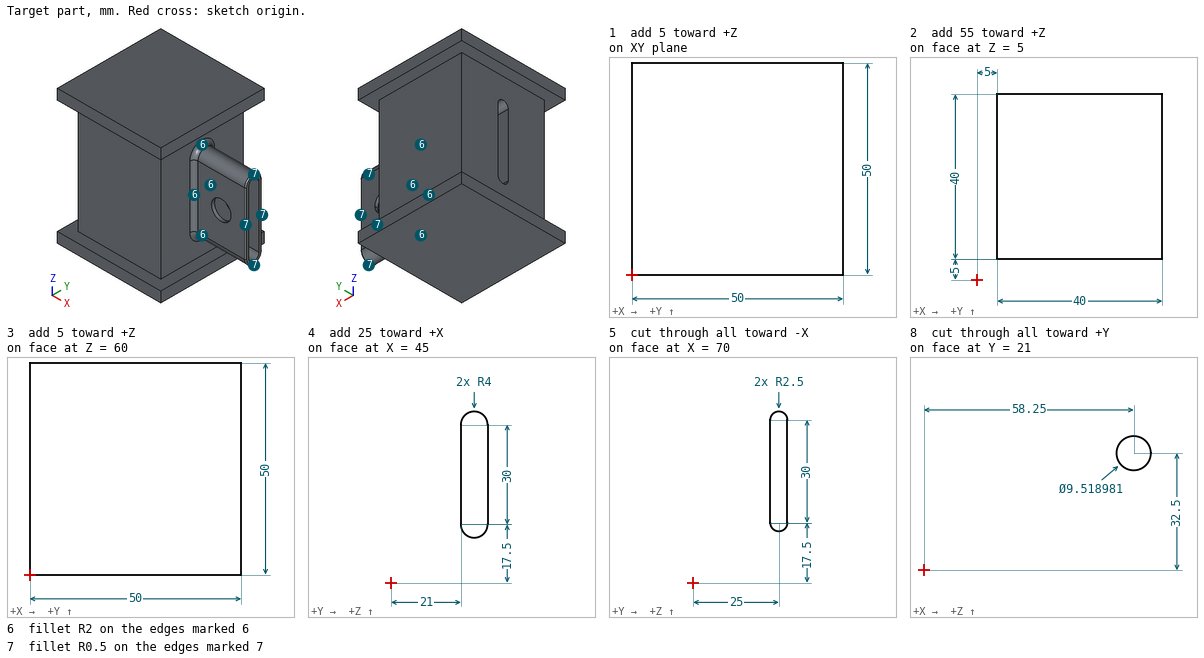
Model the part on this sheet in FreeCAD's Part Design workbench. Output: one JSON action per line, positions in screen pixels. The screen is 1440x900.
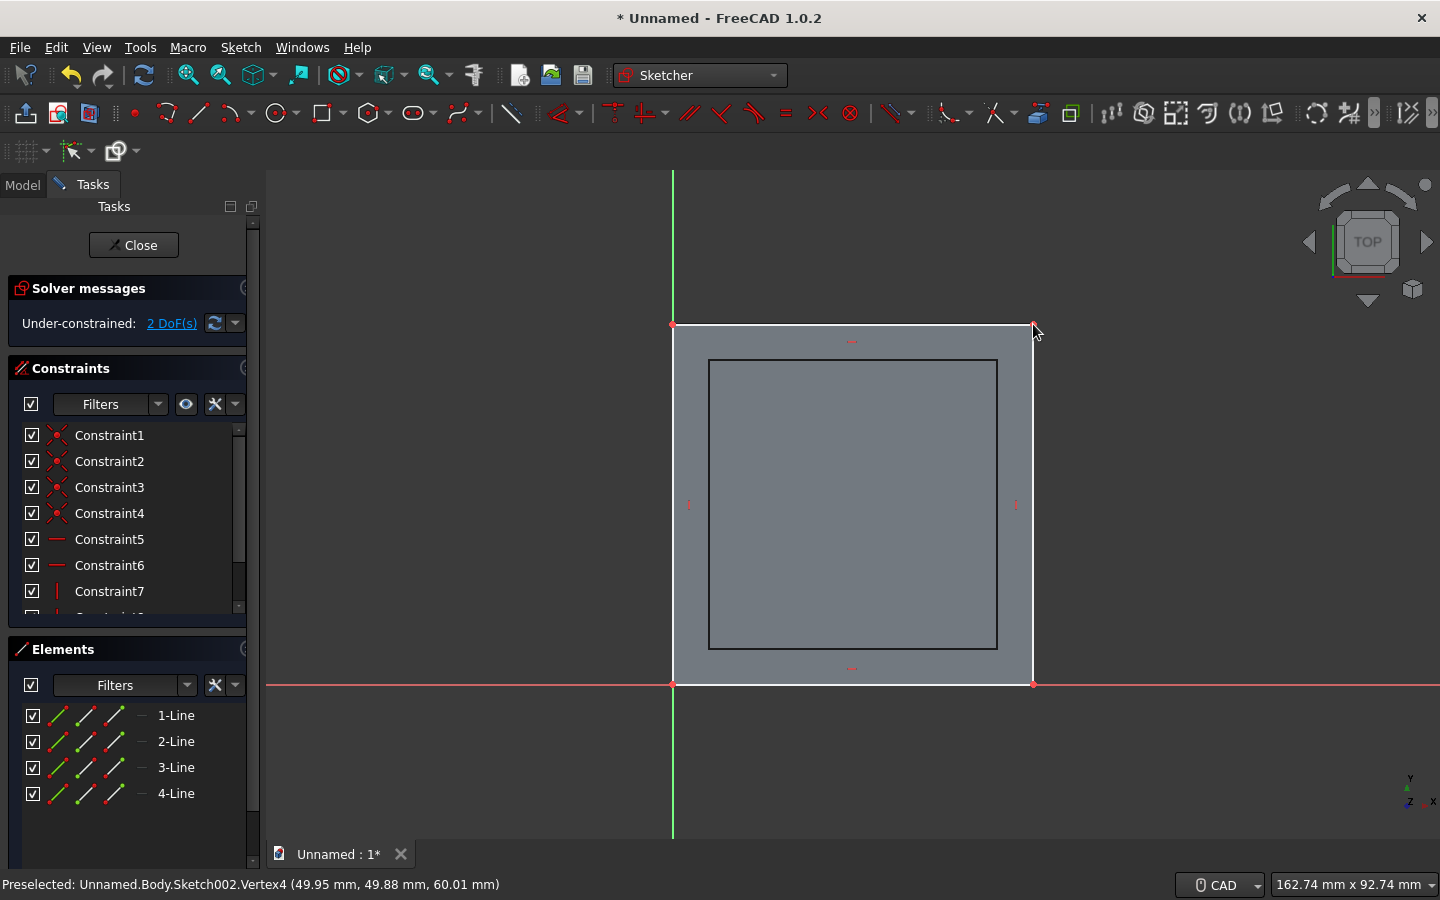
{"action": "left_click", "coordinate": [558, 114]}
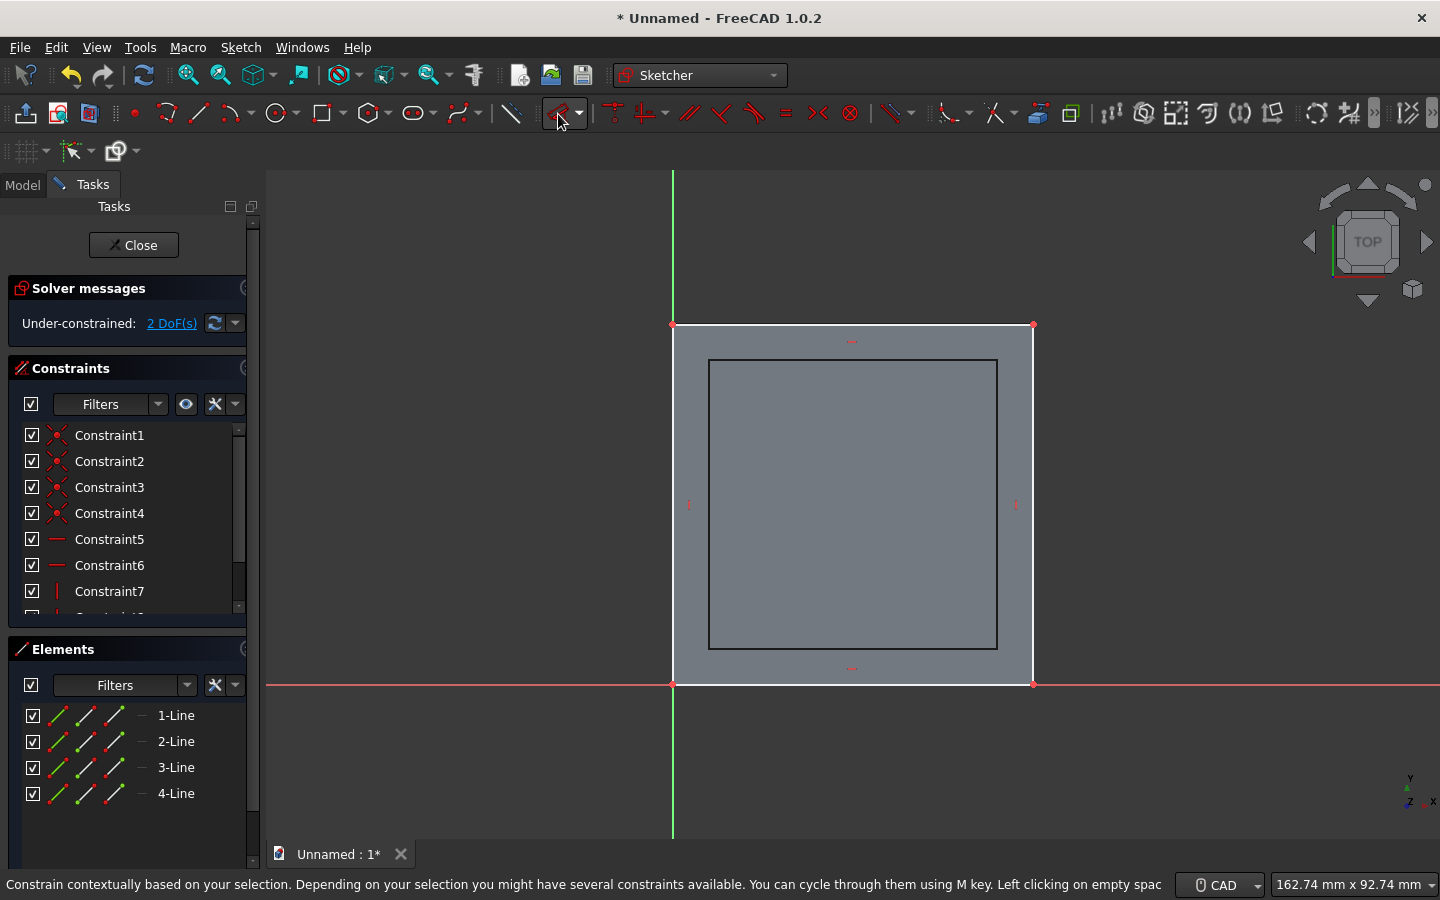
{"action": "left_click", "coordinate": [781, 685]}
{"action": "left_click", "coordinate": [853, 719]}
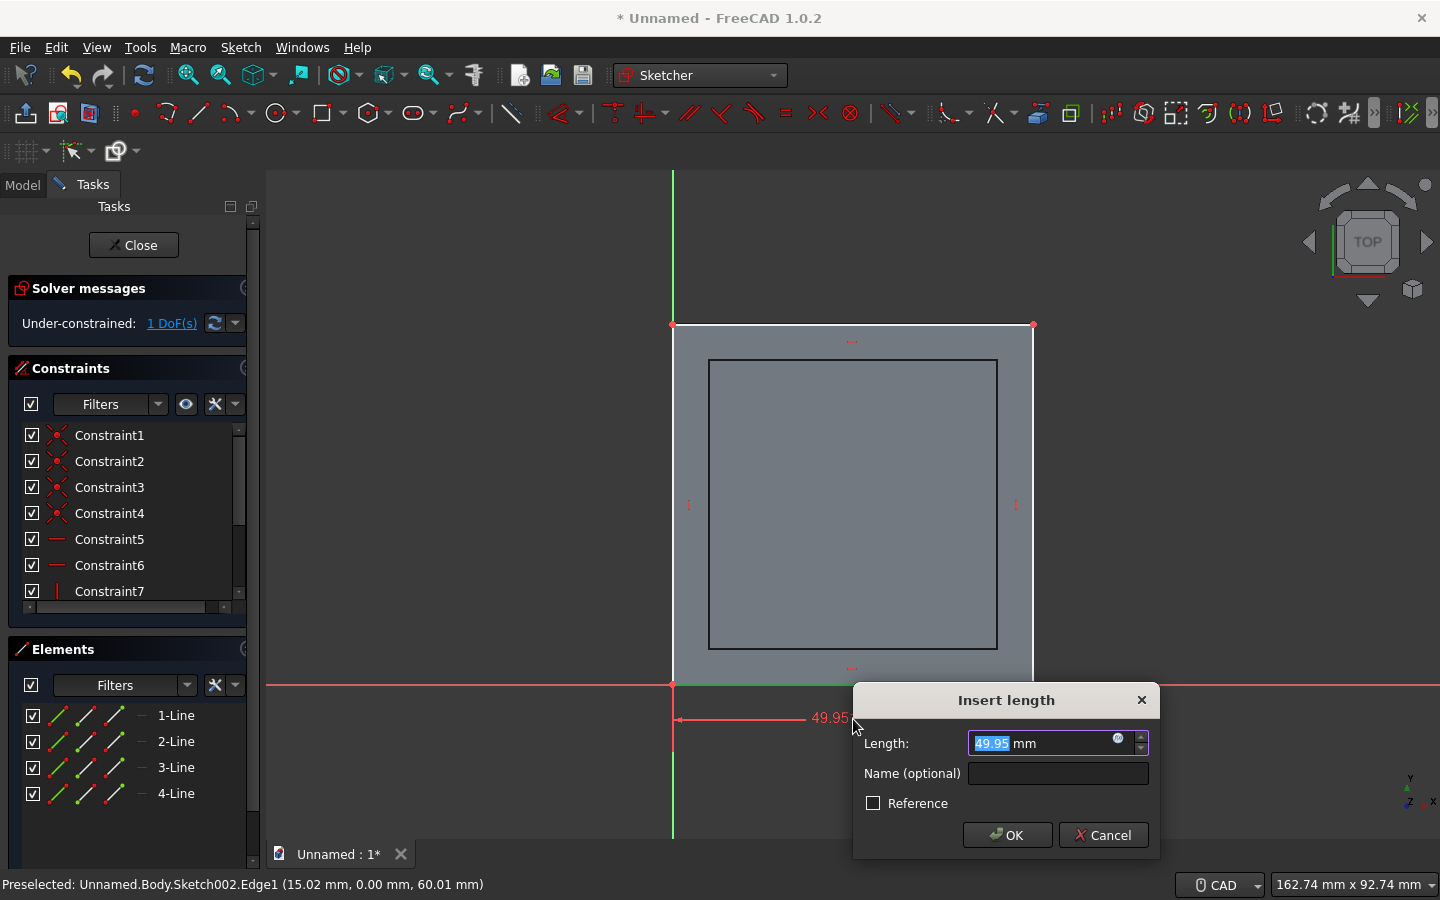
{"action": "type", "text": "50"}
{"action": "key", "text": "Return"}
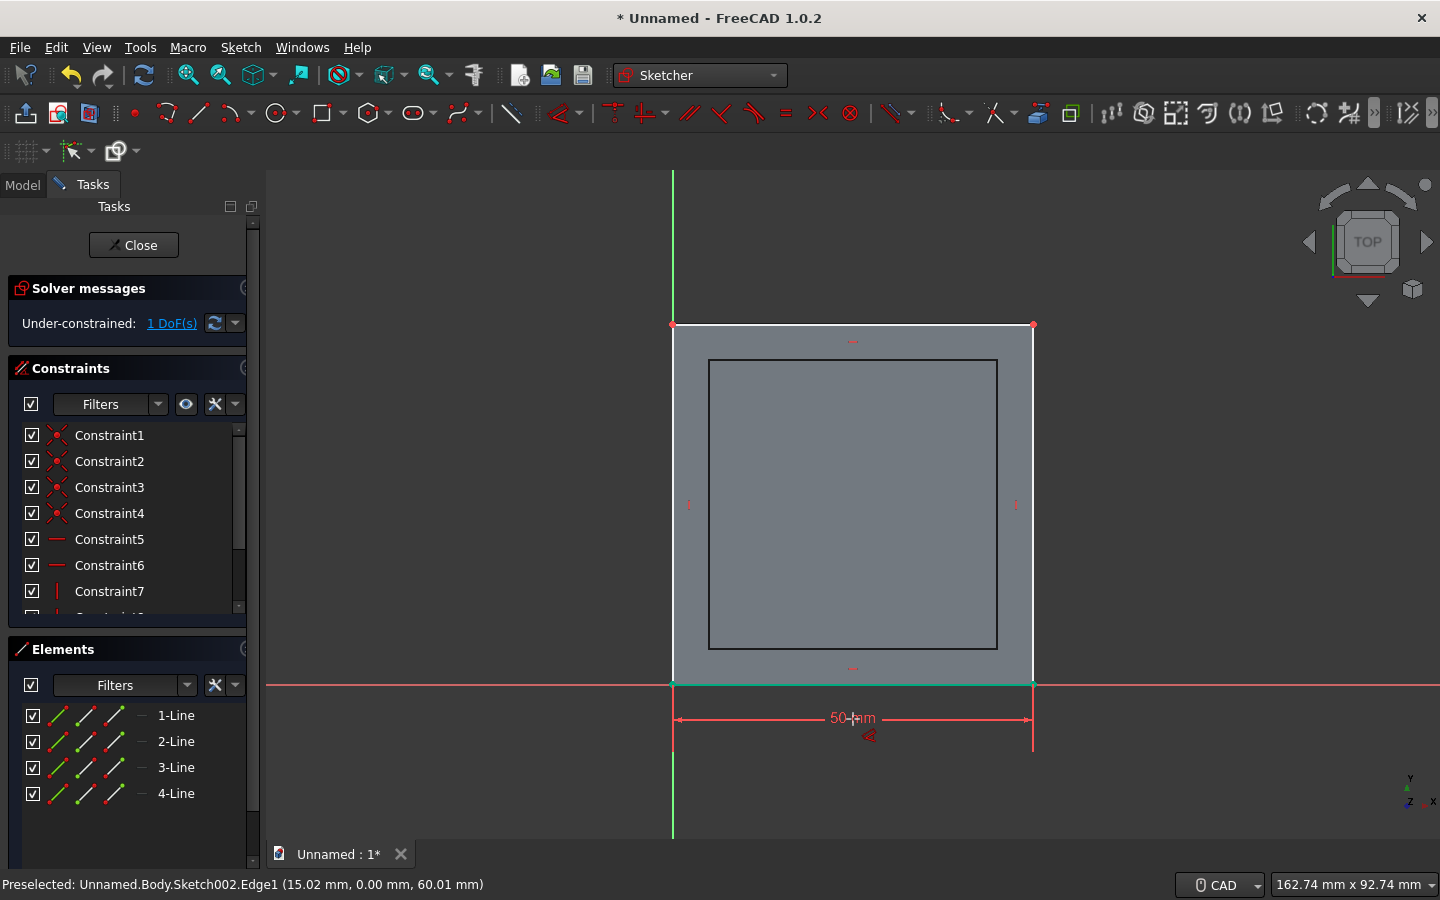
{"action": "left_click", "coordinate": [1033, 577]}
{"action": "left_click", "coordinate": [1067, 505]}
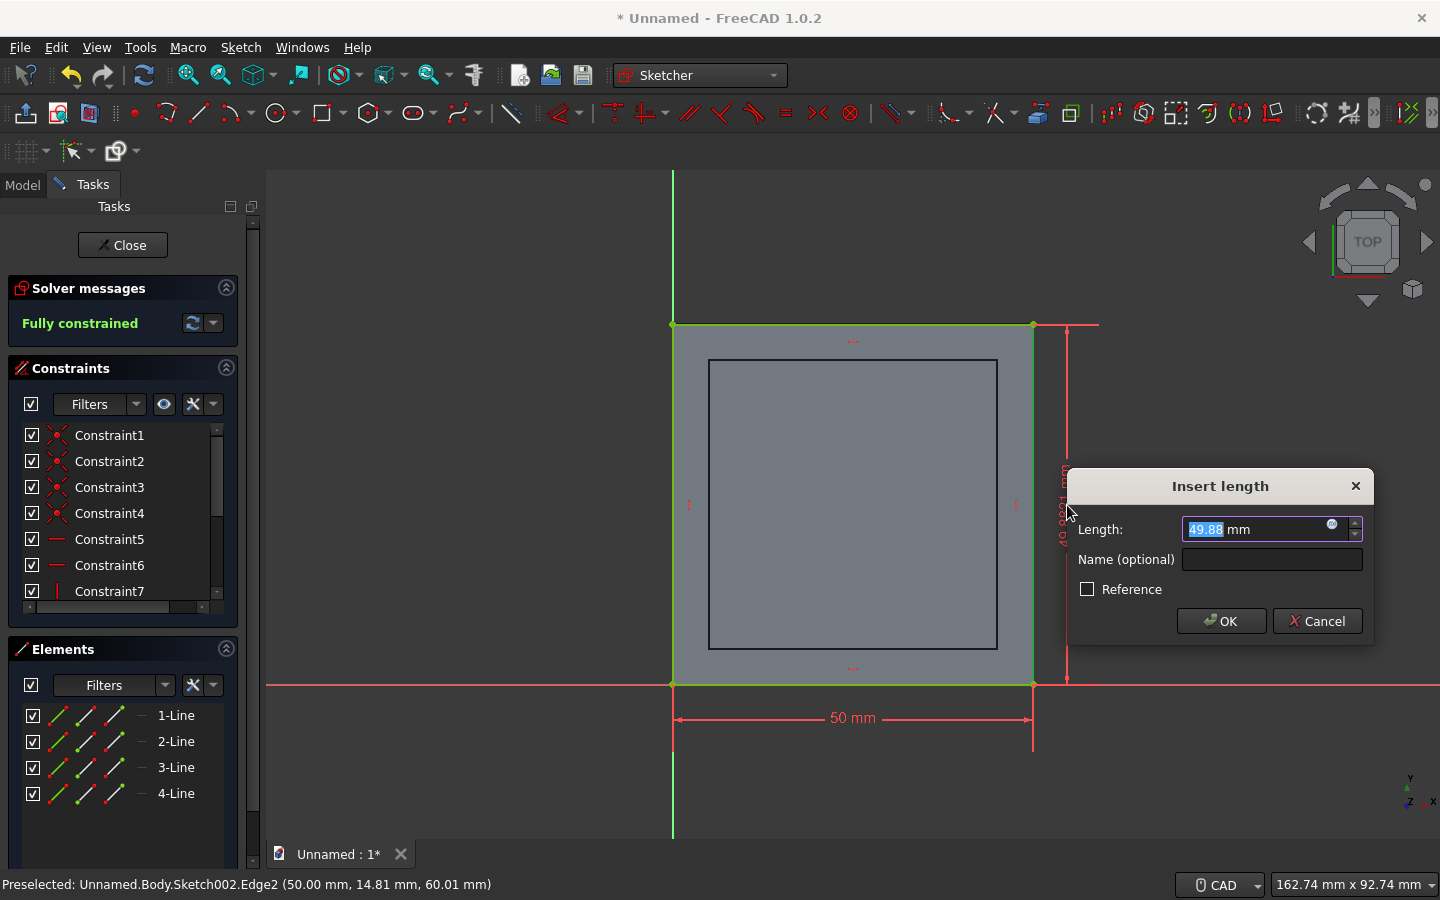
{"action": "type", "text": "50"}
{"action": "key", "text": "Return"}
{"action": "key", "text": "Escape"}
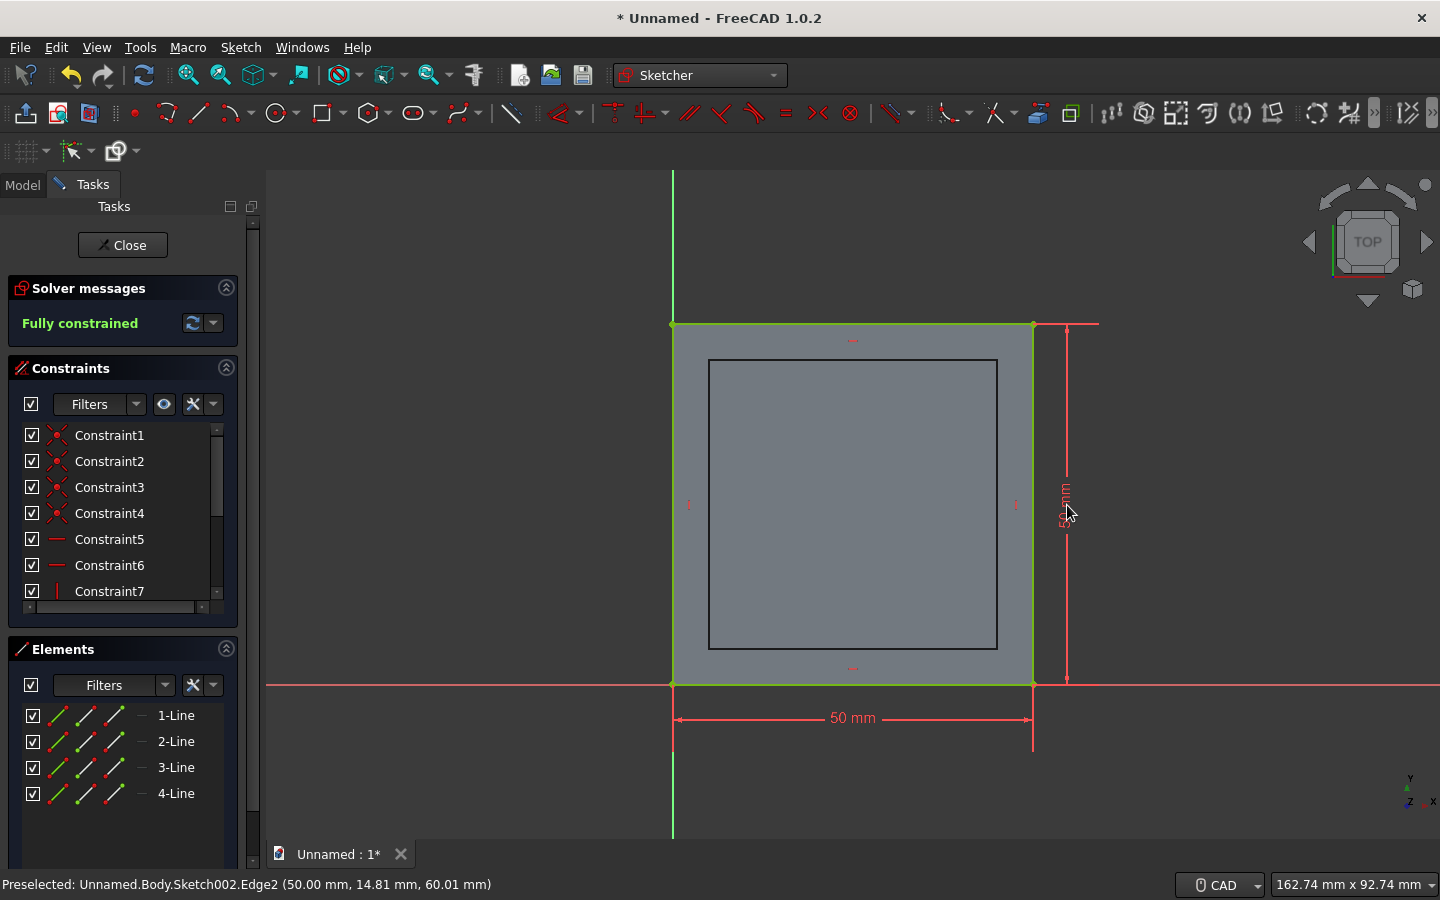
{"action": "left_click", "coordinate": [123, 245]}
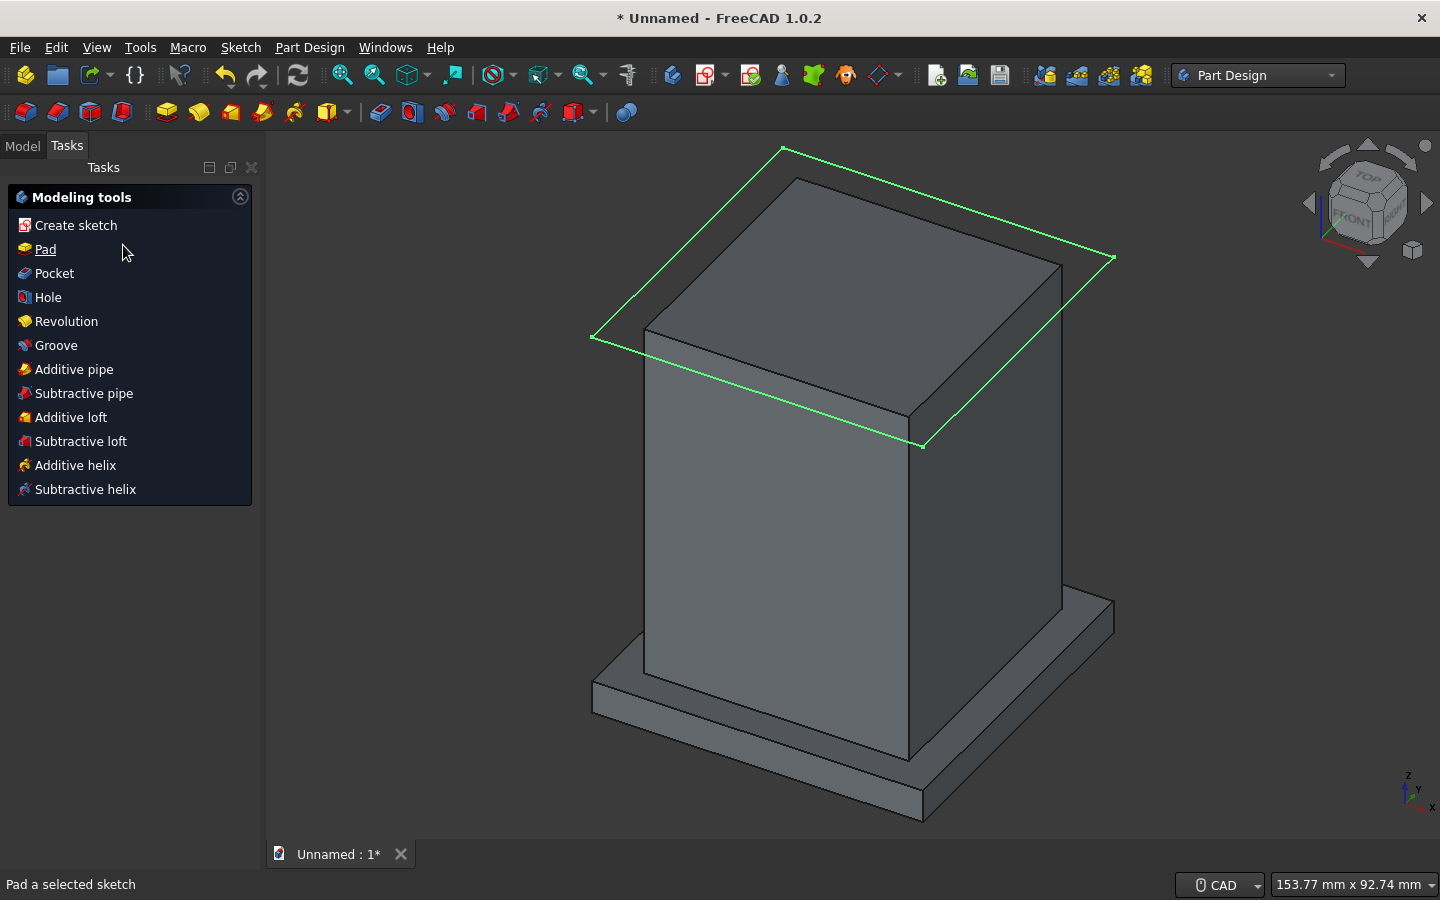
{"action": "left_click", "coordinate": [168, 112]}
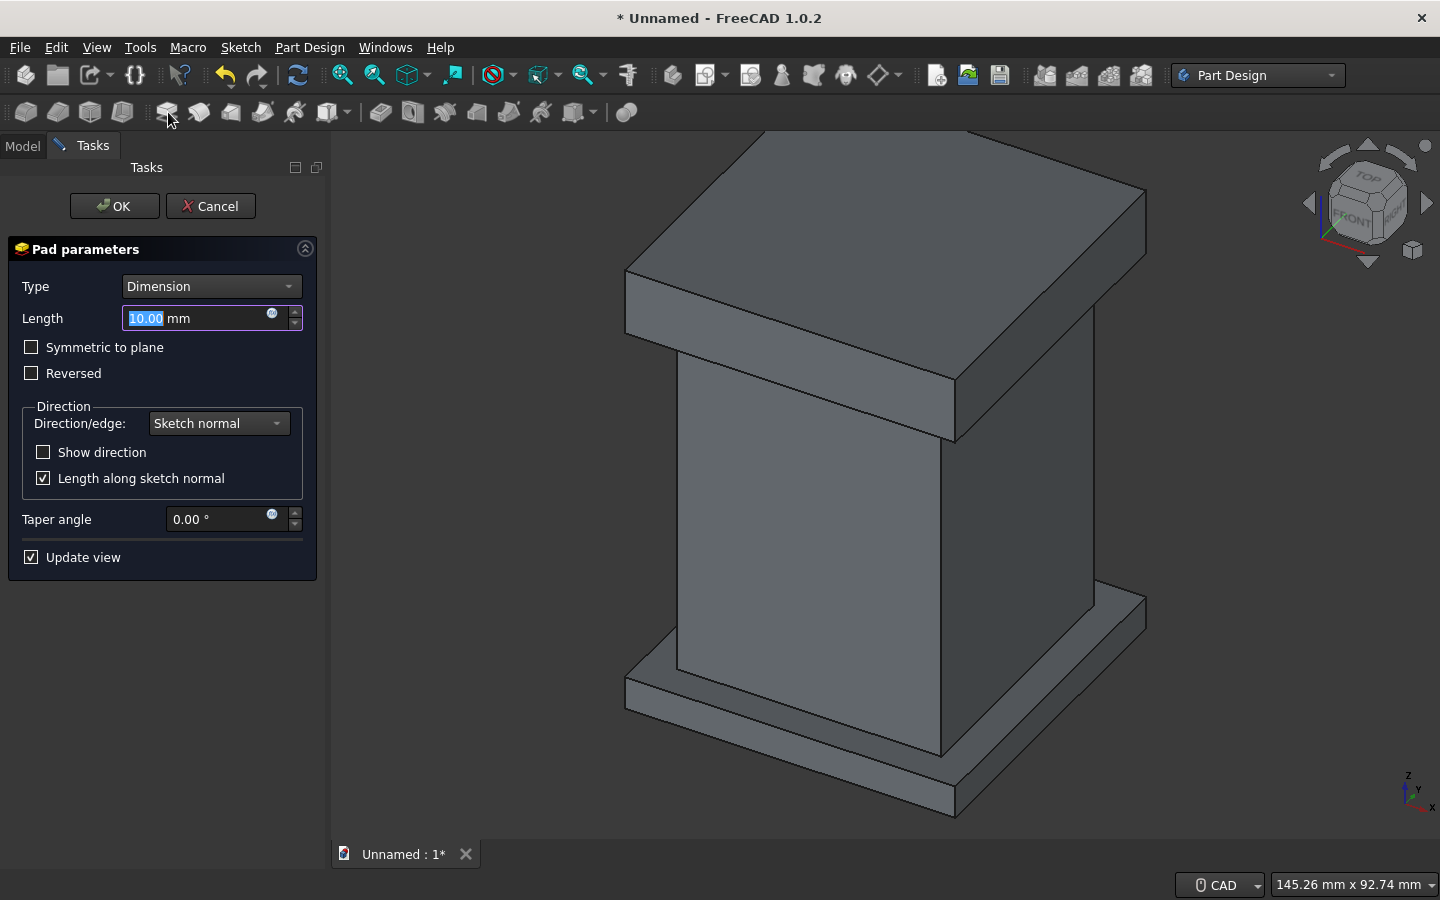
{"action": "type", "text": "5"}
{"action": "key", "text": "Tab"}